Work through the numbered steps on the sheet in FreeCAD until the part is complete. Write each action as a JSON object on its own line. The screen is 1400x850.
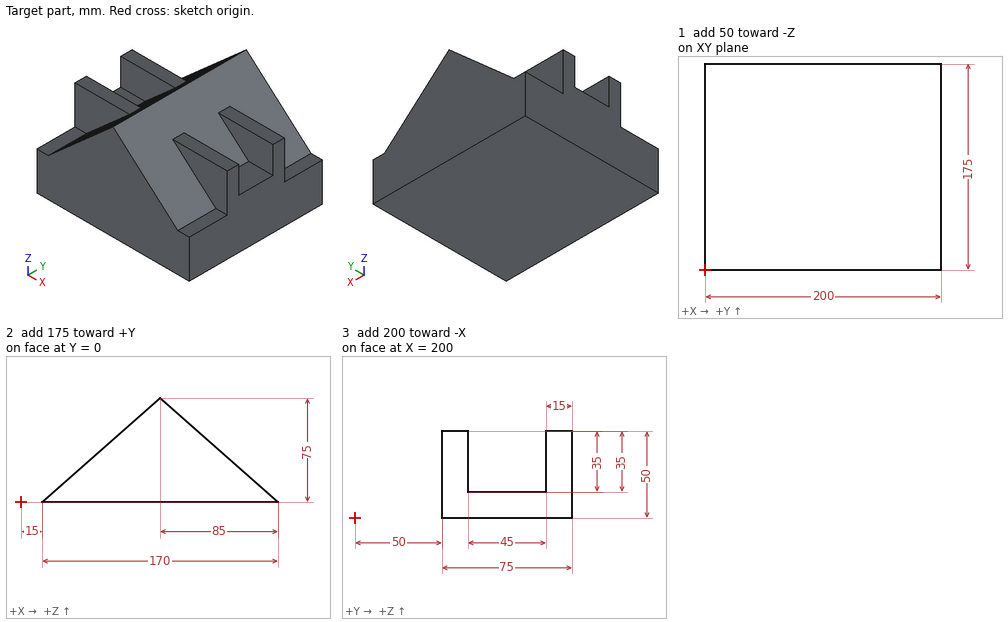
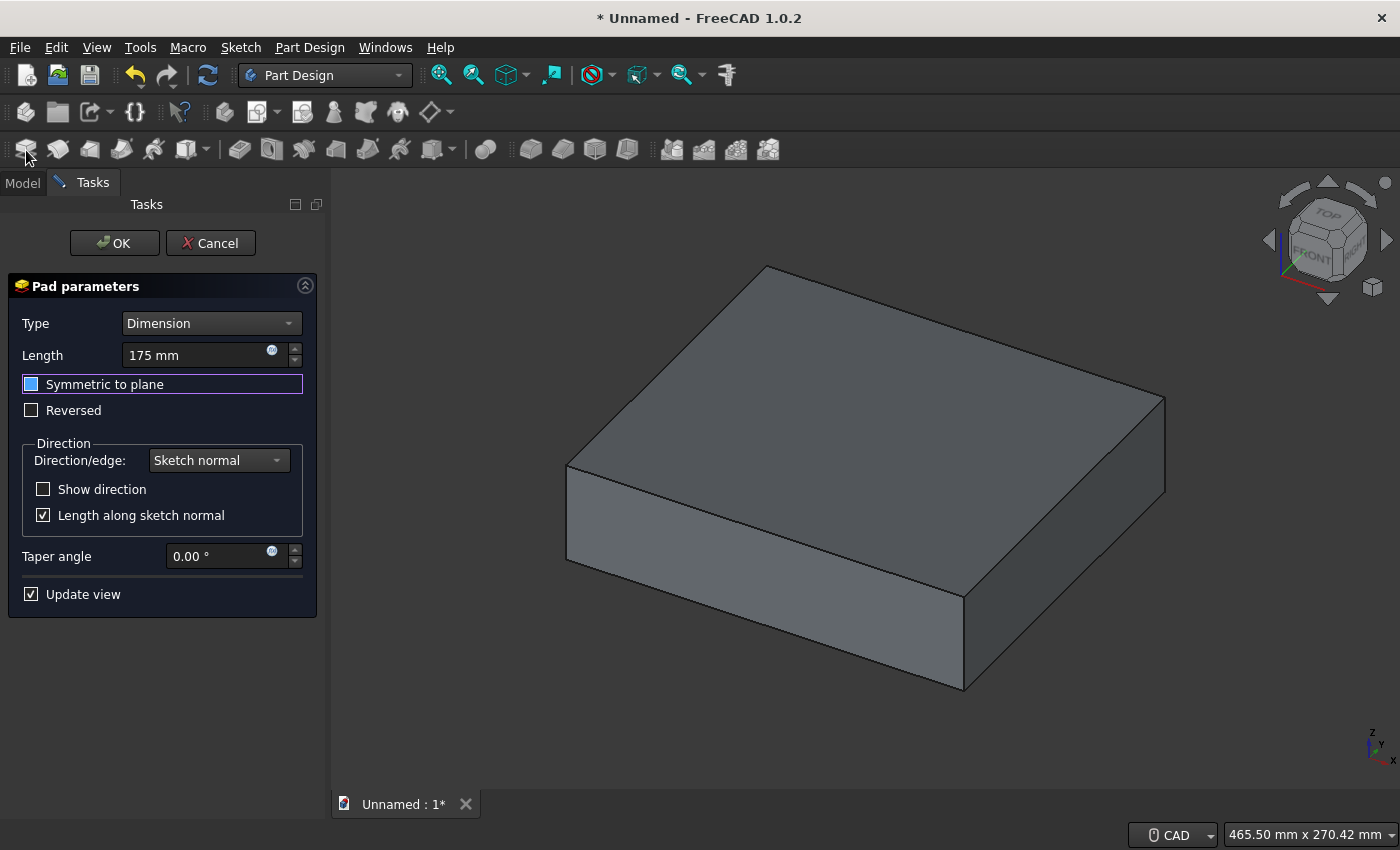
{"action": "left_click", "coordinate": [30, 410]}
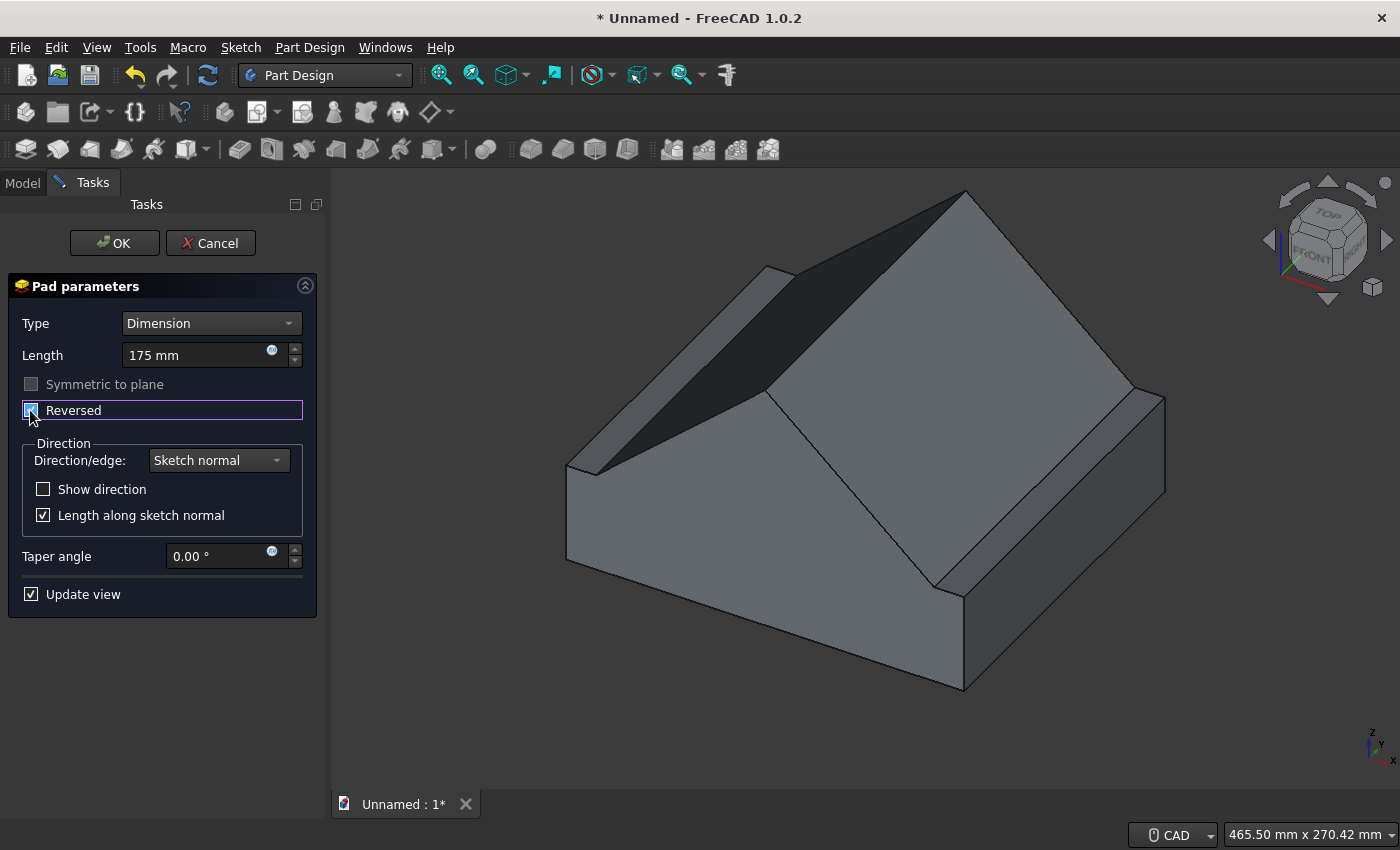
{"action": "left_click", "coordinate": [115, 243]}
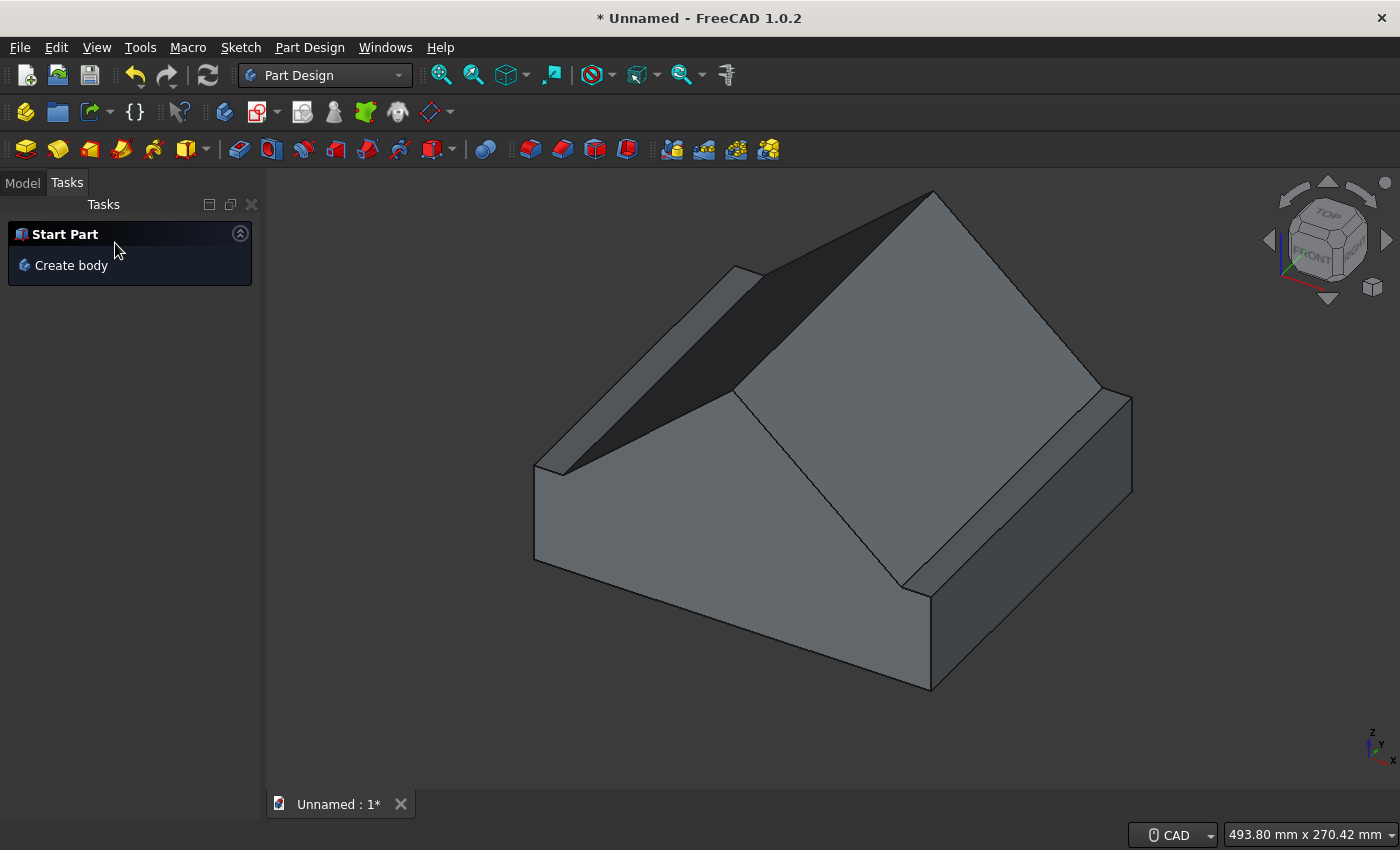
{"action": "left_click", "coordinate": [442, 76]}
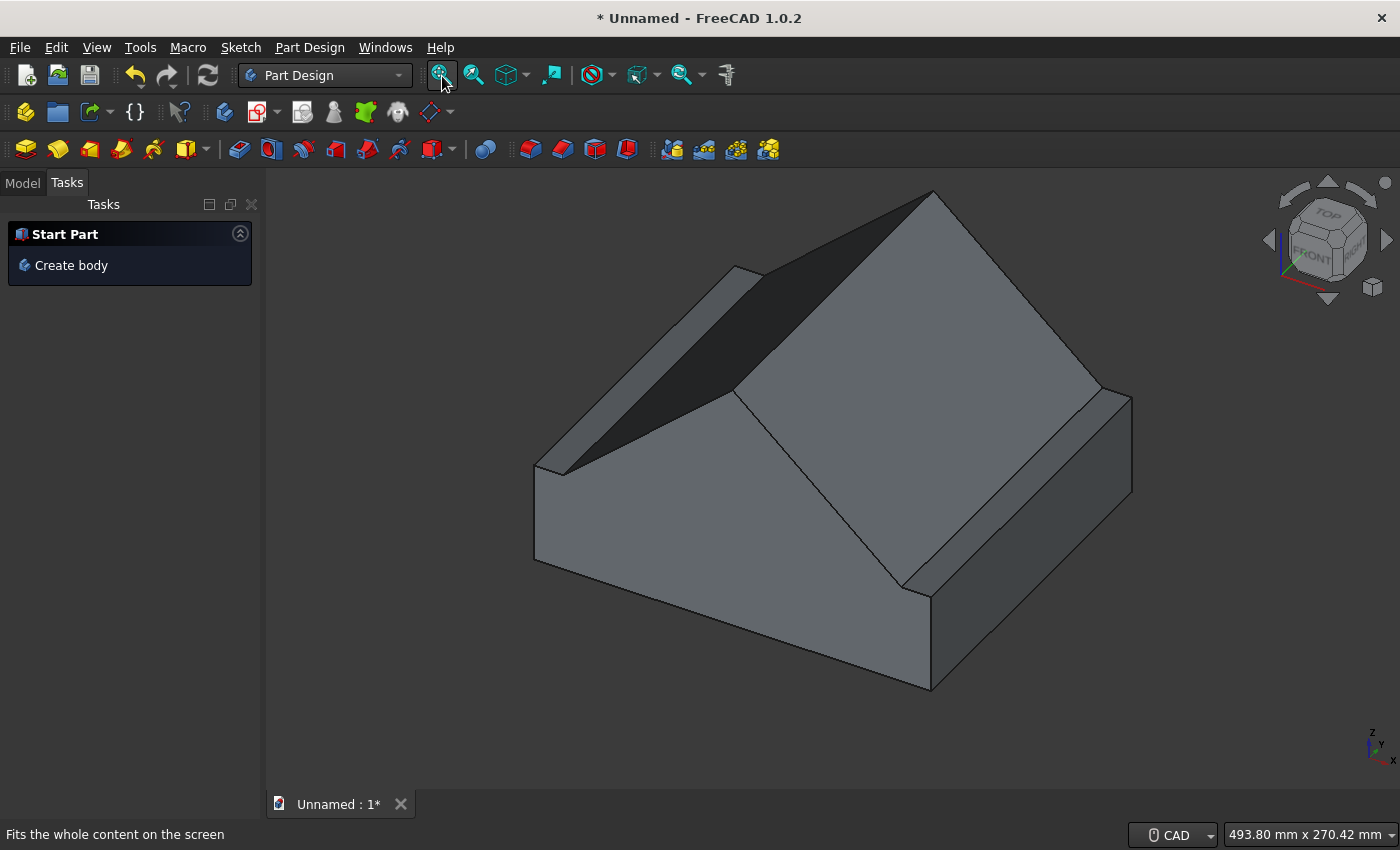
{"action": "left_click", "coordinate": [1069, 551]}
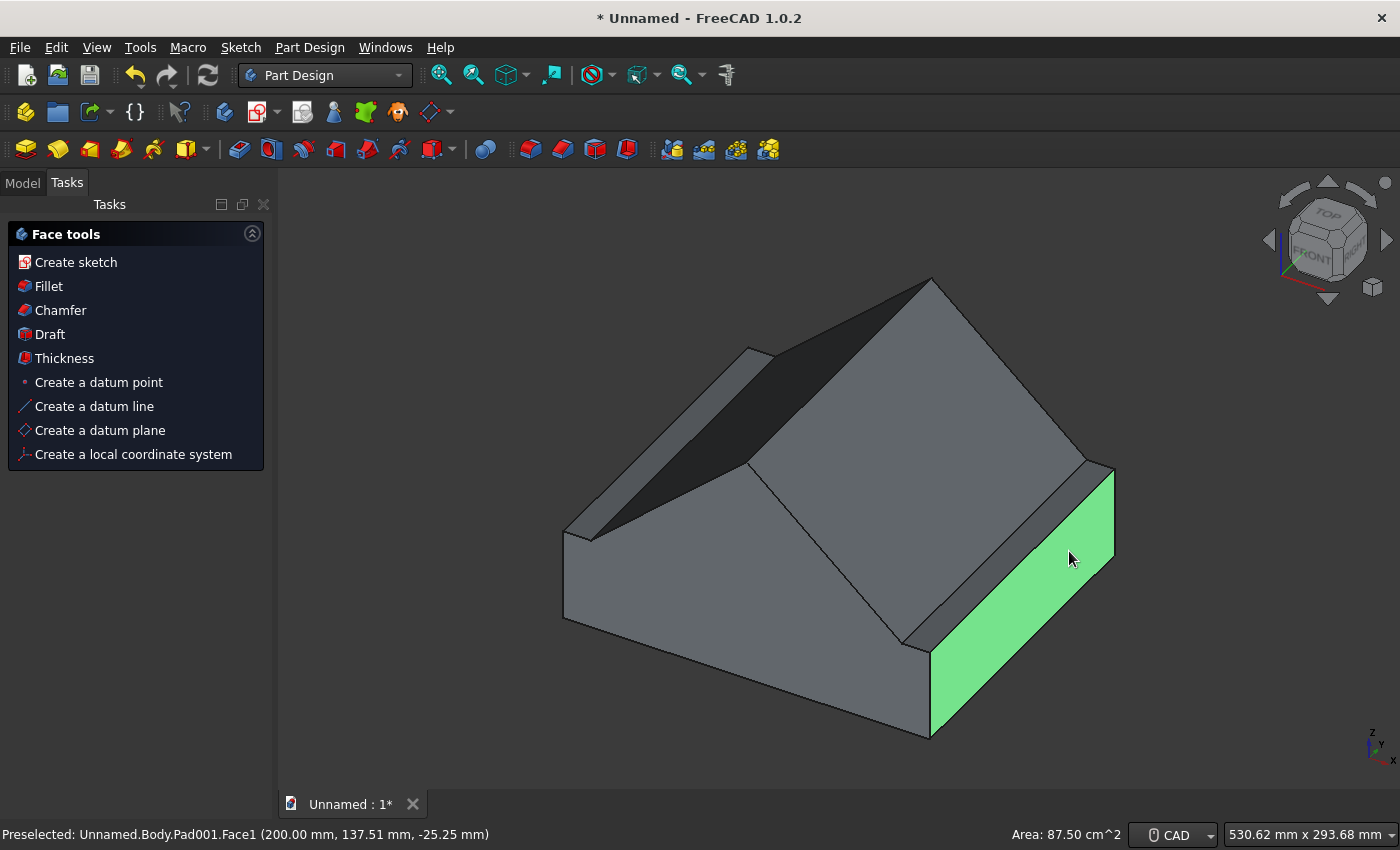
{"action": "left_click", "coordinate": [258, 112]}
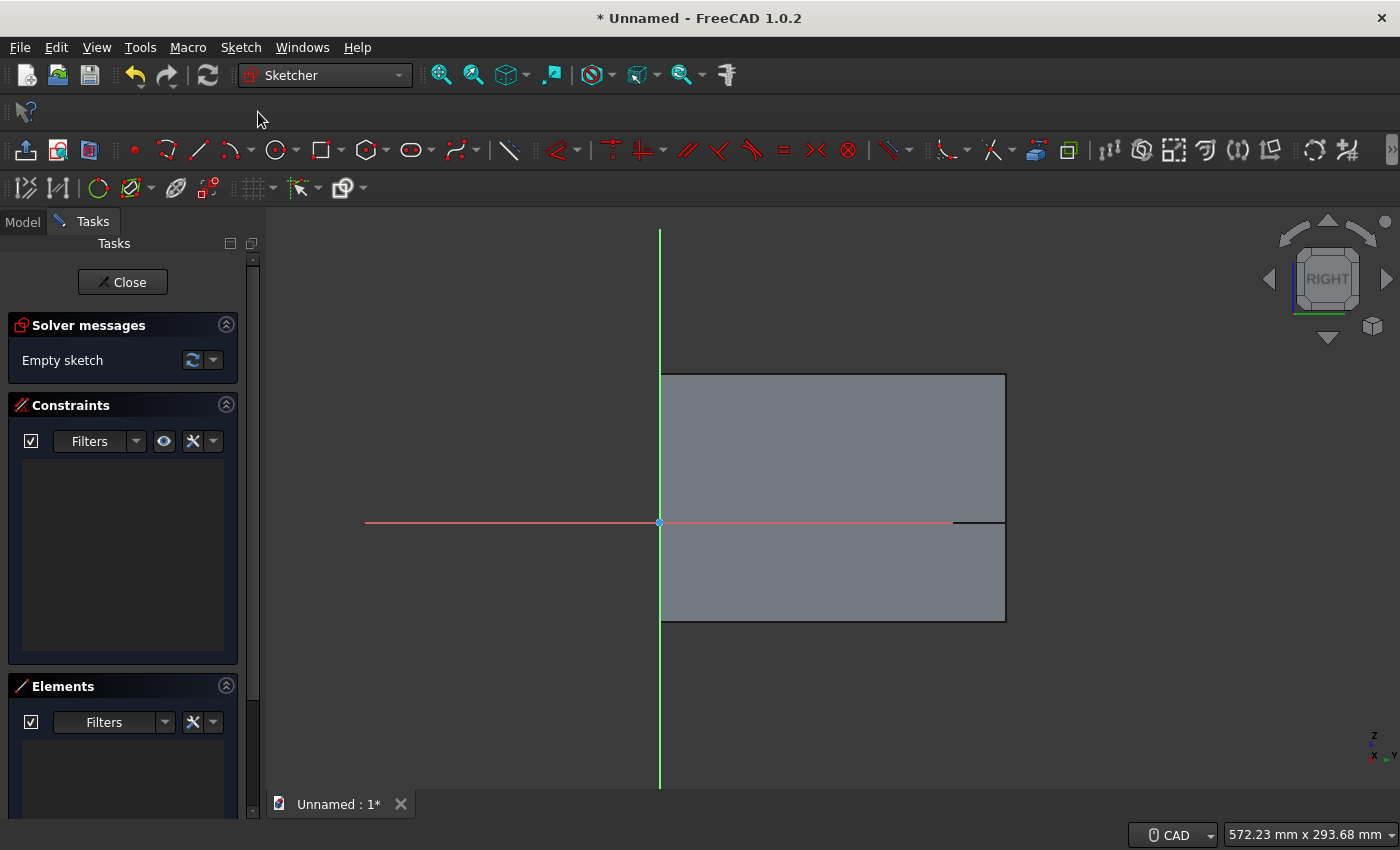
{"action": "scroll", "coordinate": [794, 459], "scroll_direction": "up", "scroll_amount": 5}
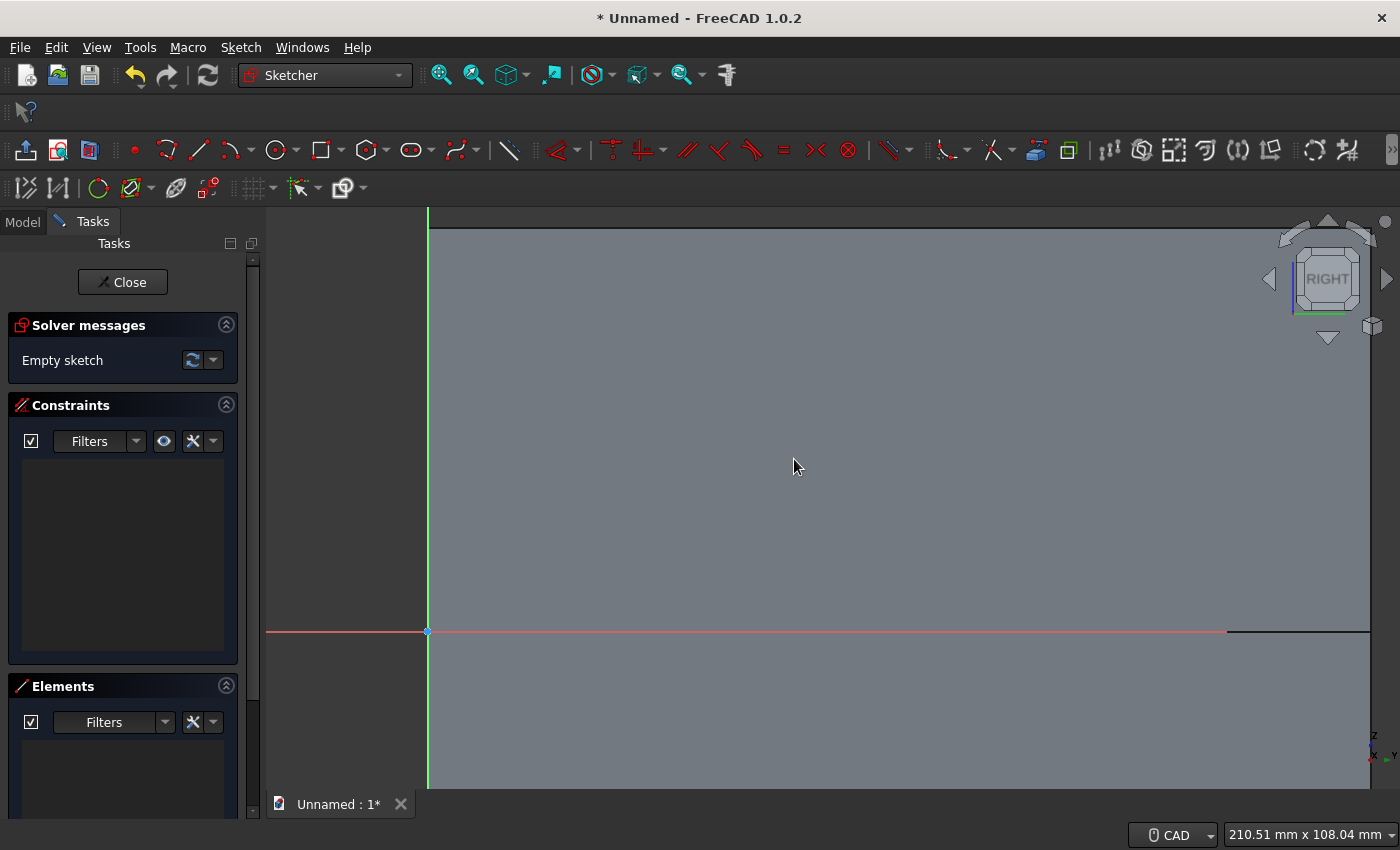
{"action": "left_click", "coordinate": [168, 150]}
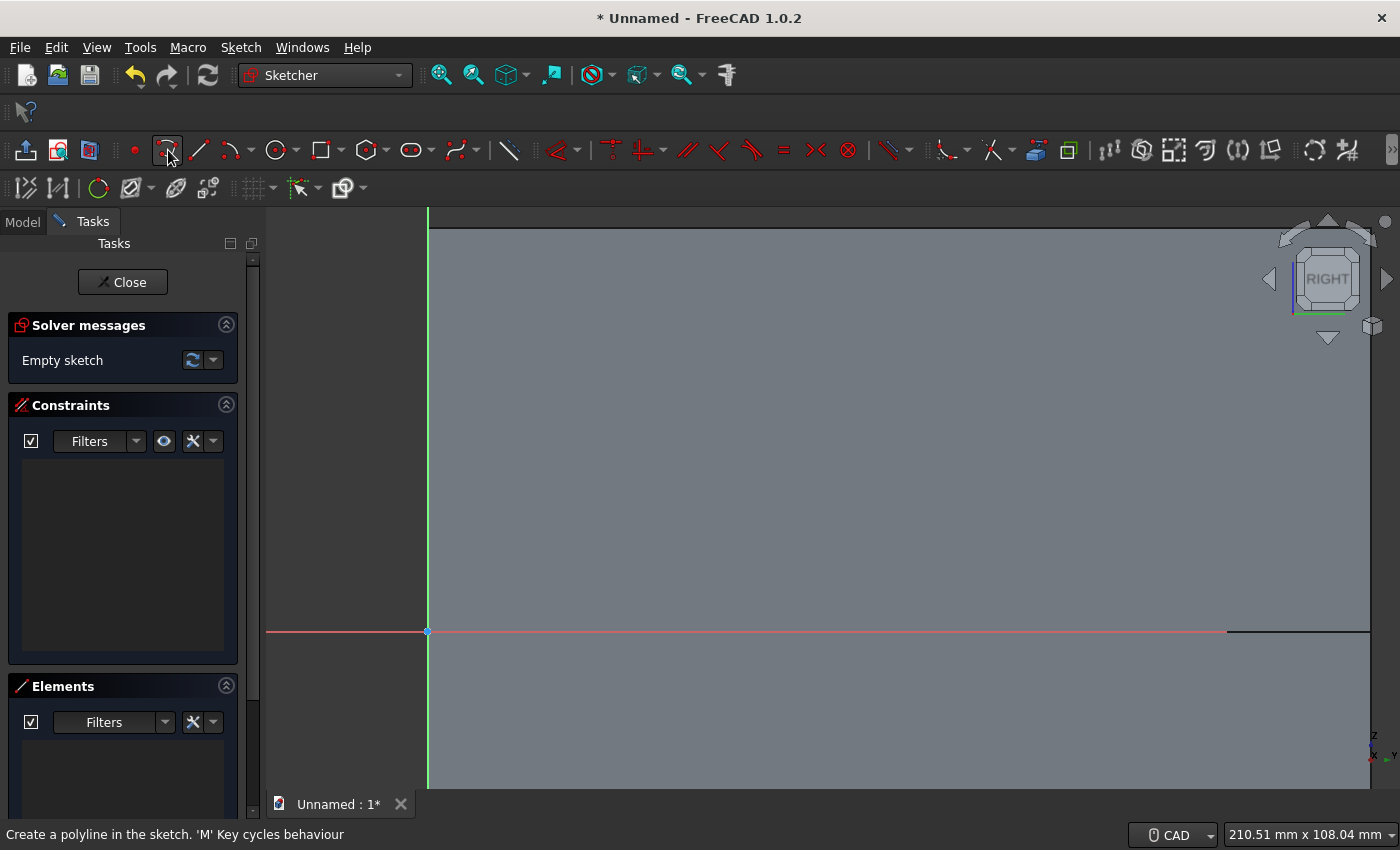
{"action": "left_click", "coordinate": [697, 632]}
{"action": "left_click", "coordinate": [1101, 623]}
{"action": "left_click", "coordinate": [1101, 362]}
{"action": "left_click", "coordinate": [1020, 362]}
{"action": "left_click", "coordinate": [1020, 551]}
{"action": "left_click", "coordinate": [778, 551]}
{"action": "left_click", "coordinate": [778, 362]}
{"action": "left_click", "coordinate": [697, 362]}
{"action": "left_click", "coordinate": [697, 632]}
{"action": "key", "text": "Escape"}
{"action": "key", "text": "Escape"}